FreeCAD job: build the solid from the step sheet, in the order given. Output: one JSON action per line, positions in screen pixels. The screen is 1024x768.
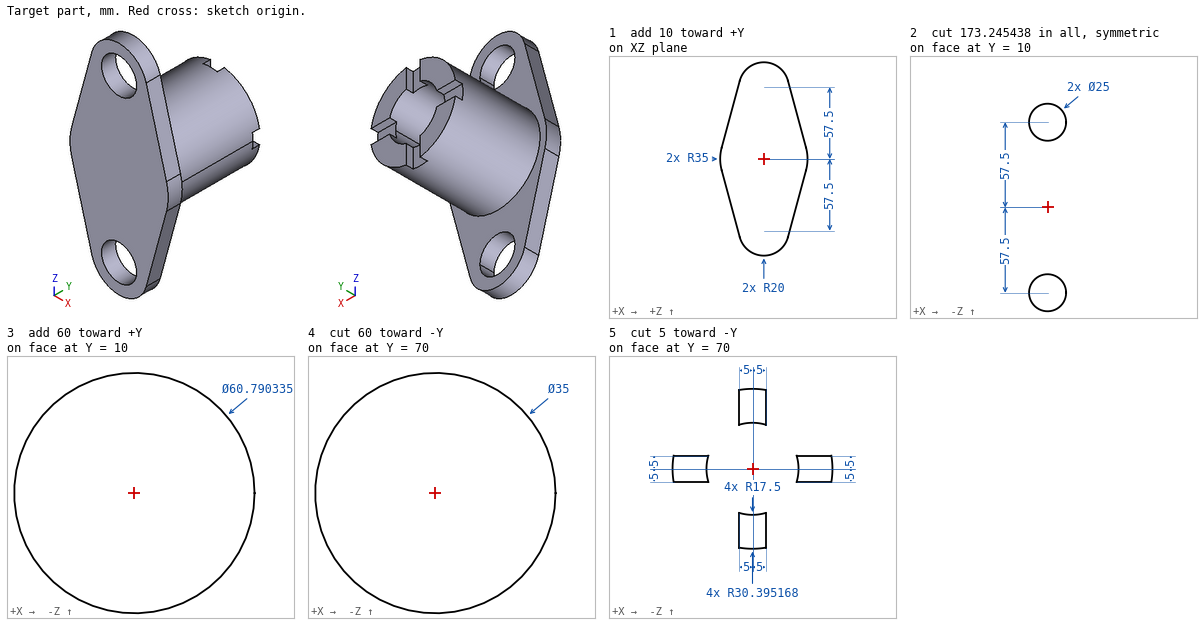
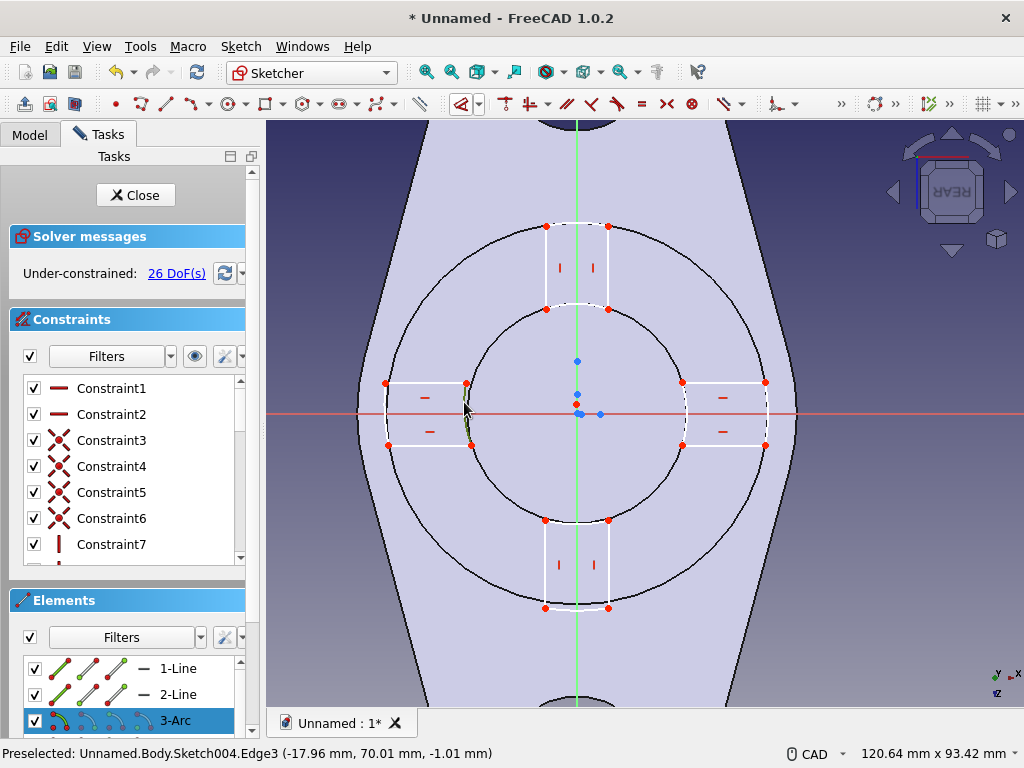
{"action": "left_click", "coordinate": [590, 305]}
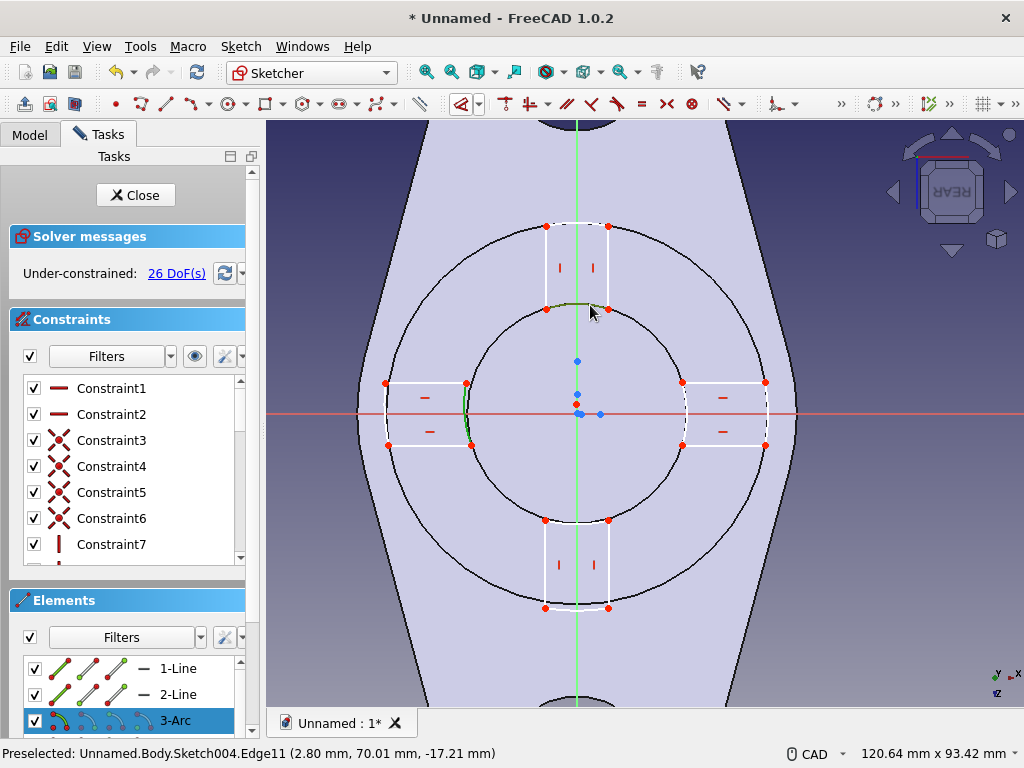
{"action": "left_click", "coordinate": [505, 104]}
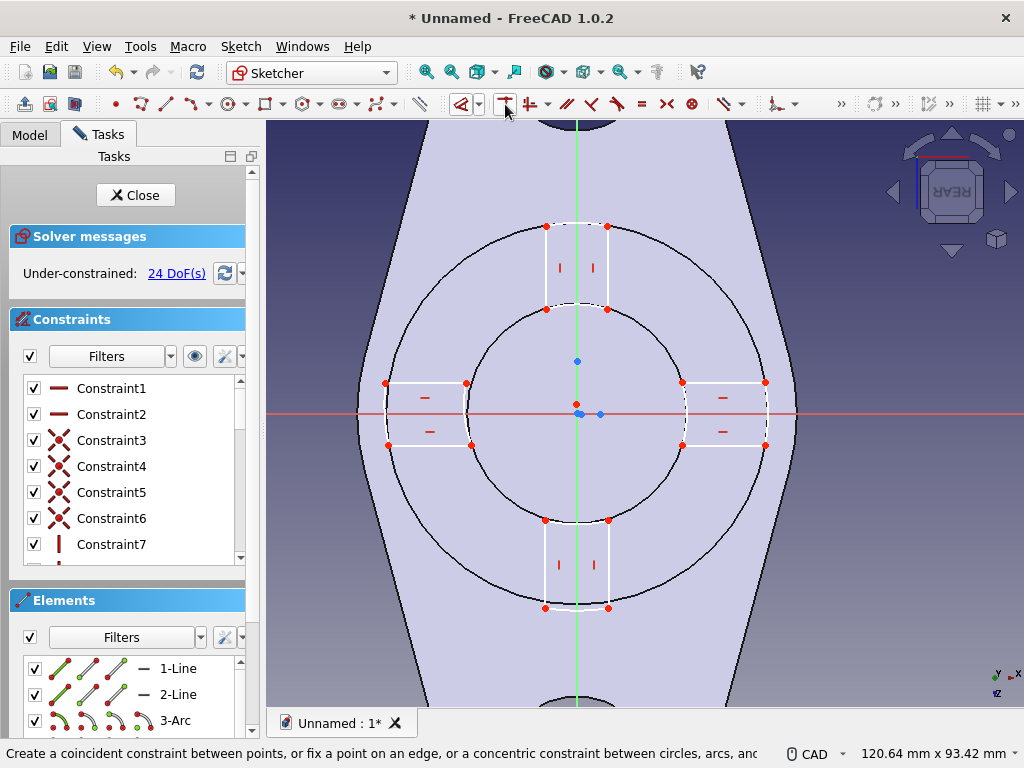
{"action": "left_click", "coordinate": [464, 402]}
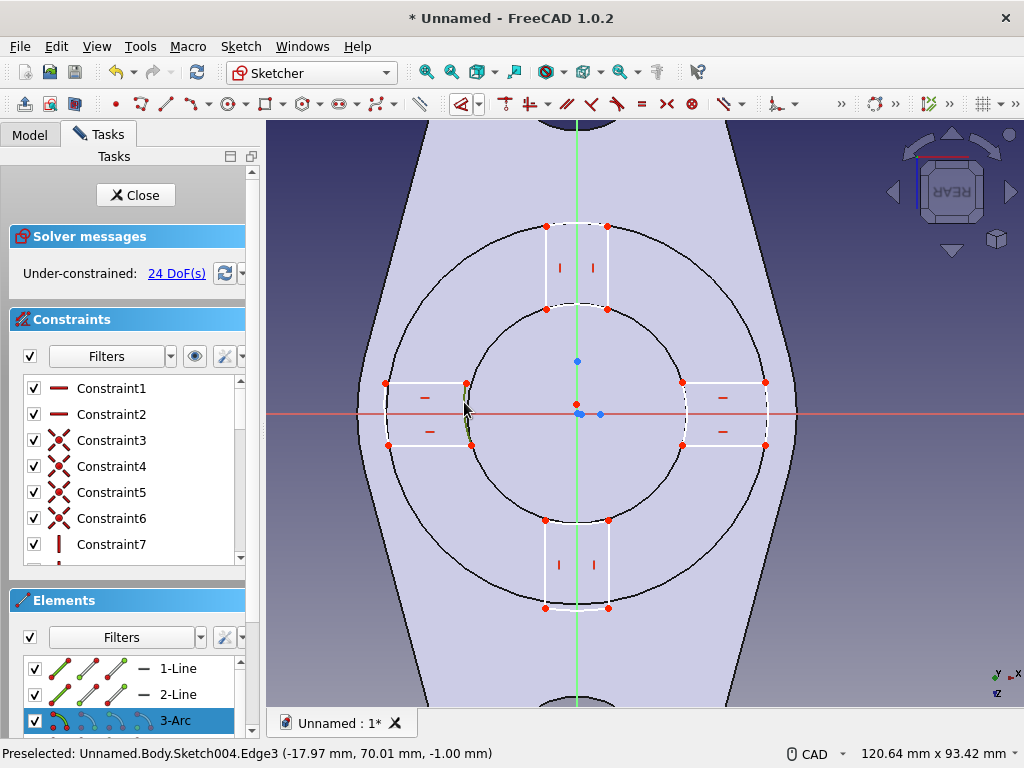
{"action": "left_click", "coordinate": [589, 223]}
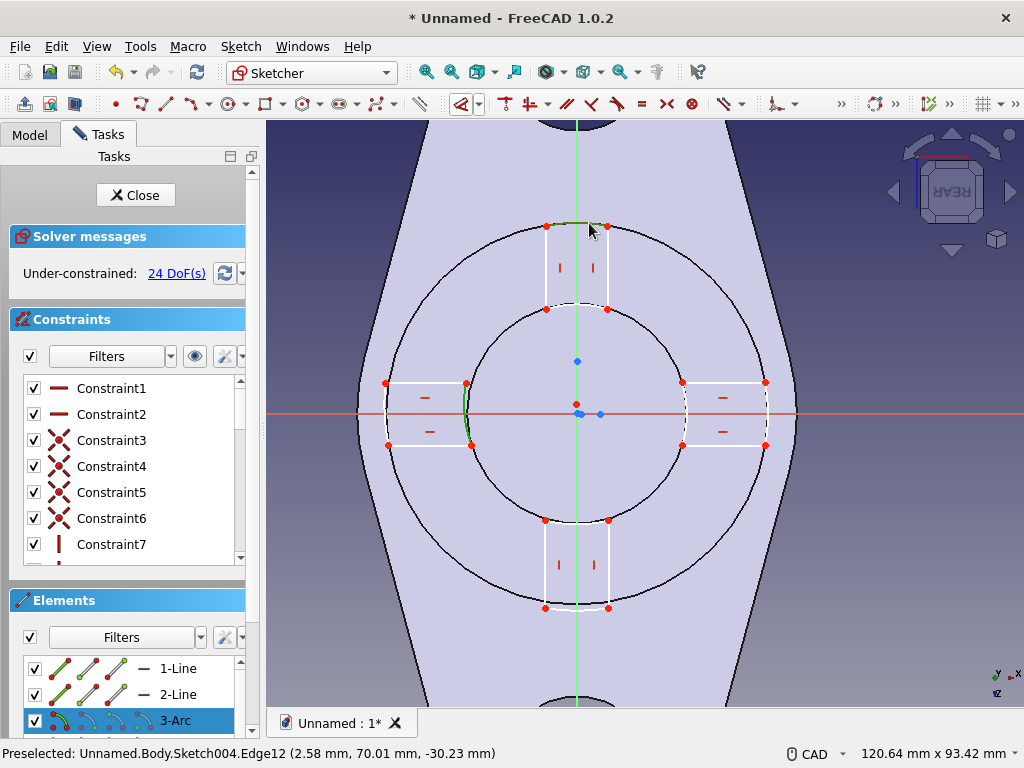
{"action": "left_click", "coordinate": [505, 104]}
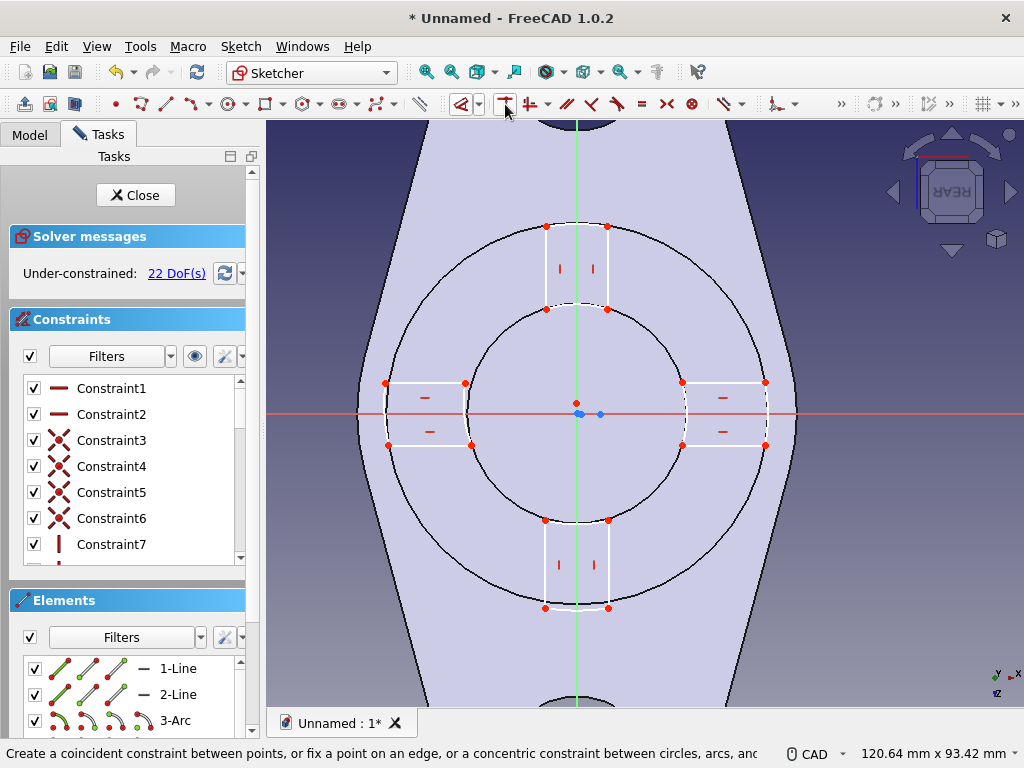
{"action": "left_click", "coordinate": [464, 402]}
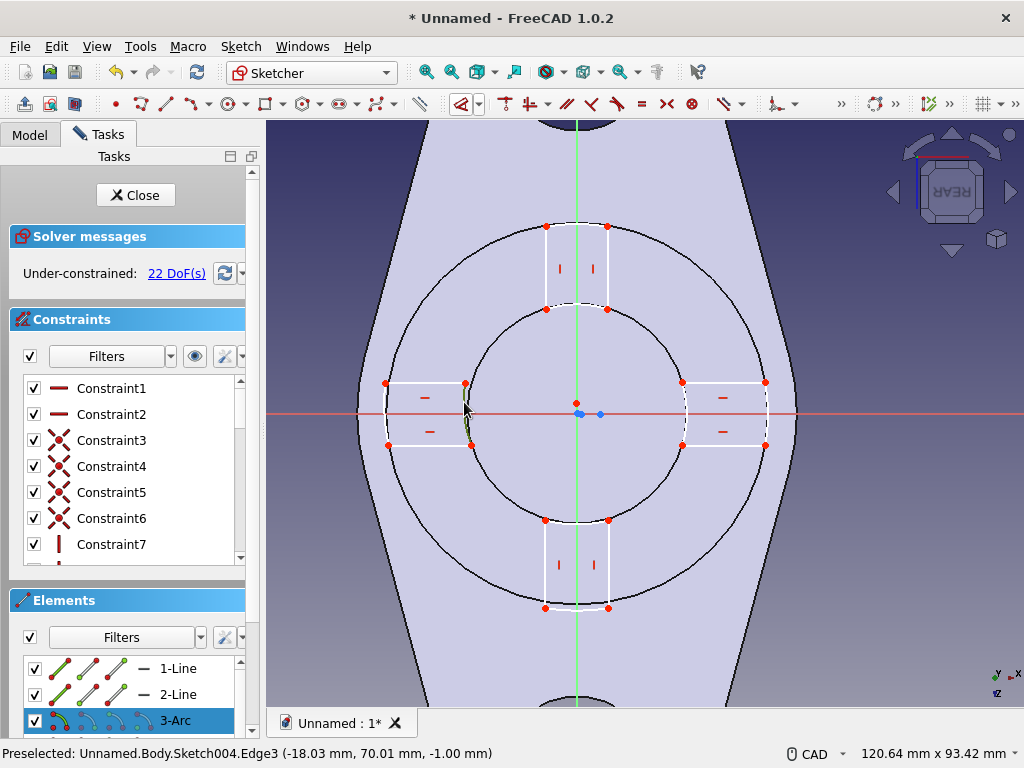
{"action": "left_click", "coordinate": [686, 427]}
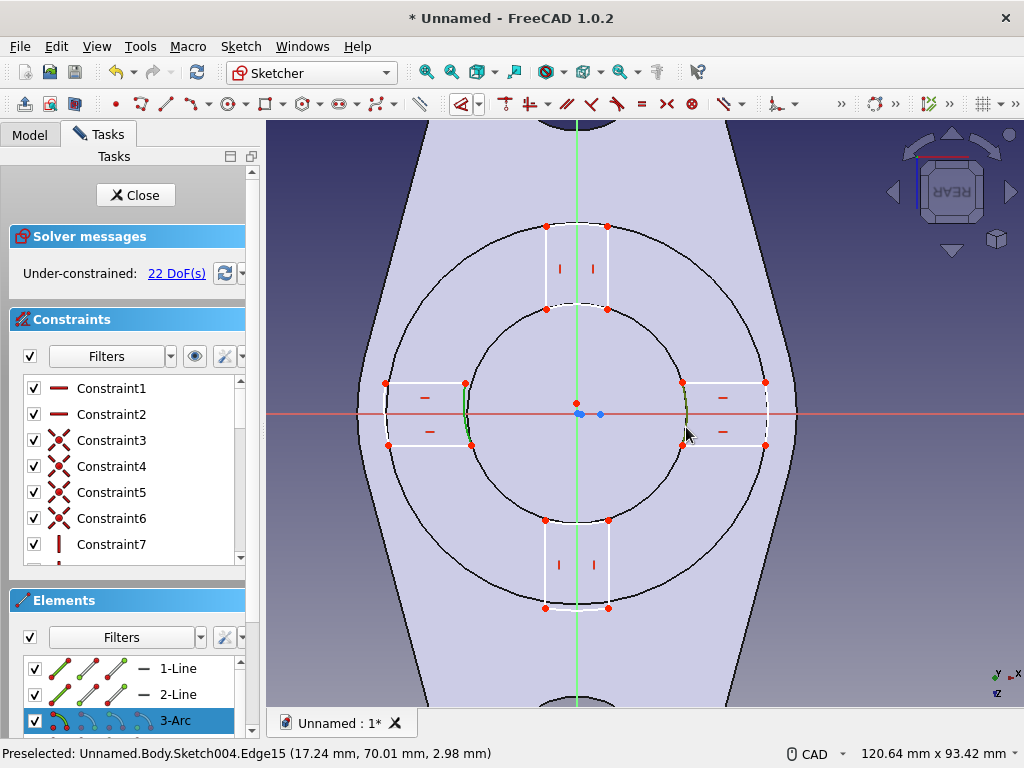
{"action": "left_click", "coordinate": [505, 104]}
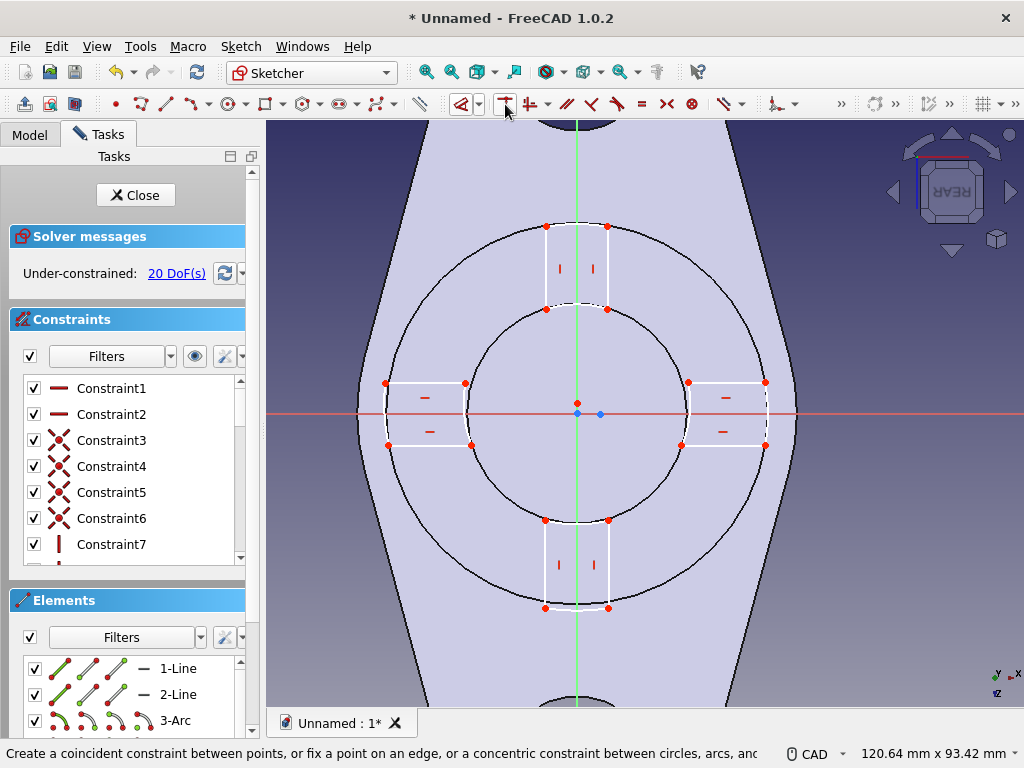
{"action": "left_click", "coordinate": [464, 402]}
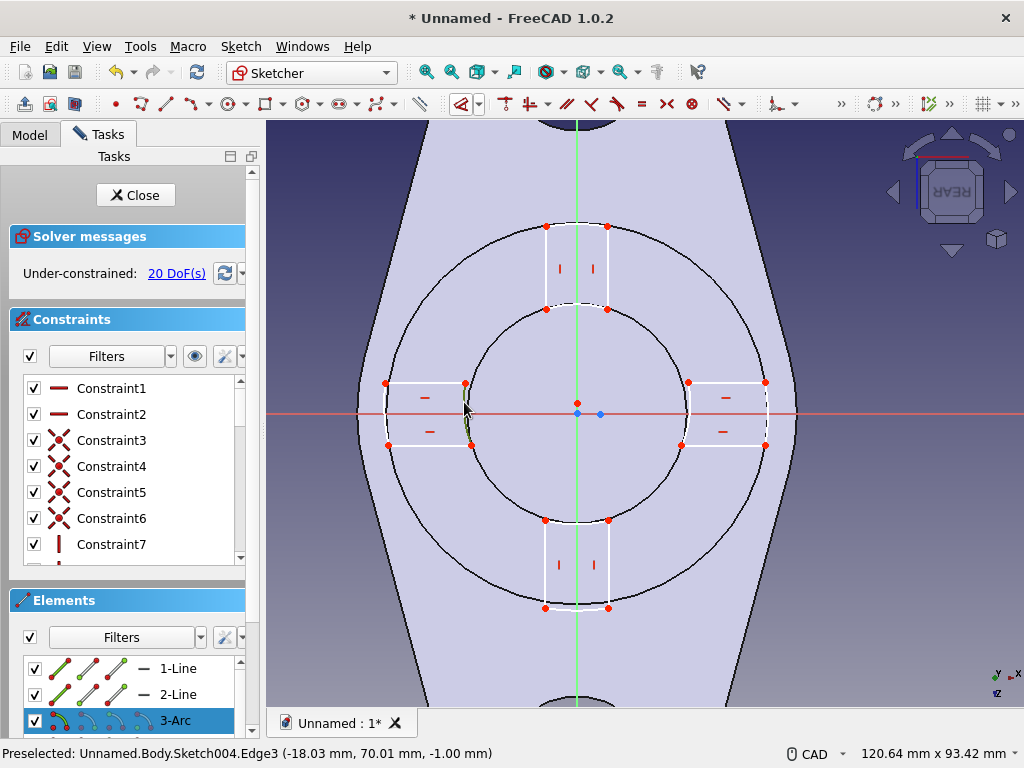
{"action": "left_click", "coordinate": [768, 427]}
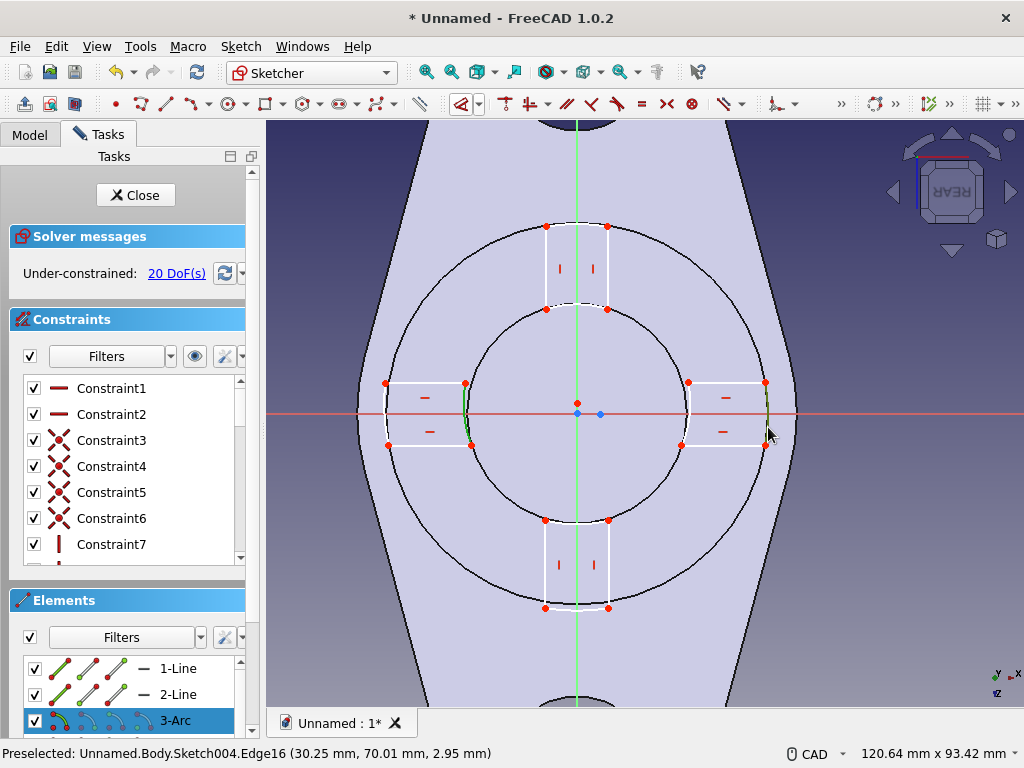
{"action": "left_click", "coordinate": [505, 104]}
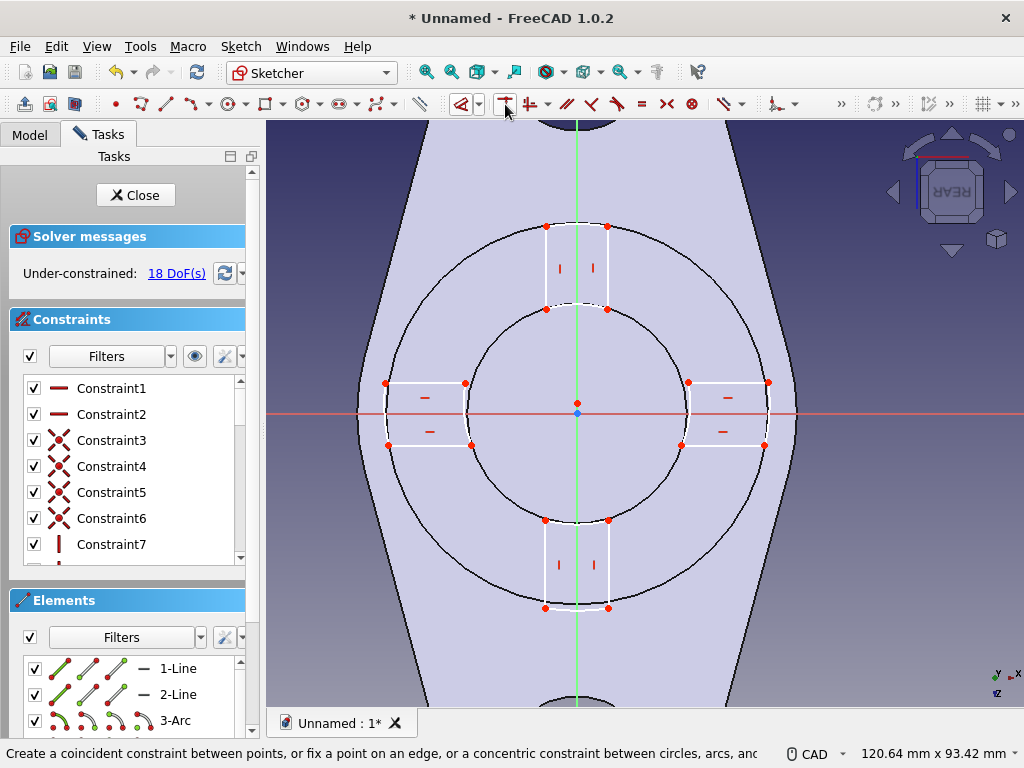
{"action": "left_click_drag", "start_coordinate": [567, 394], "coordinate": [587, 424]}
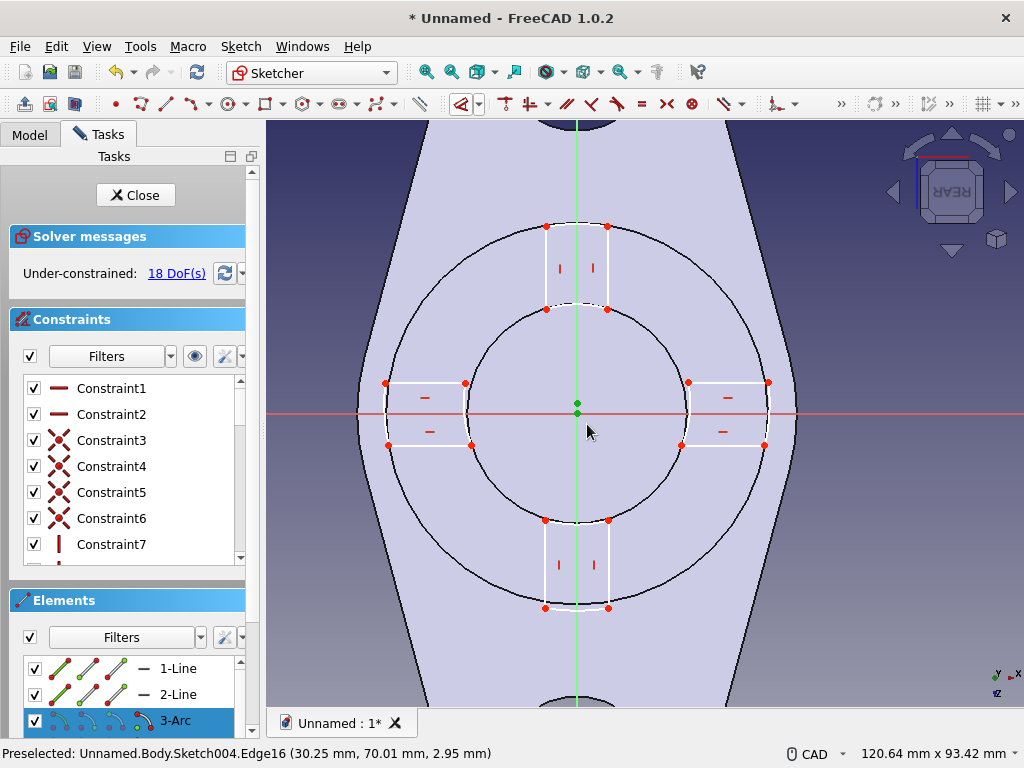
{"action": "left_click", "coordinate": [505, 104]}